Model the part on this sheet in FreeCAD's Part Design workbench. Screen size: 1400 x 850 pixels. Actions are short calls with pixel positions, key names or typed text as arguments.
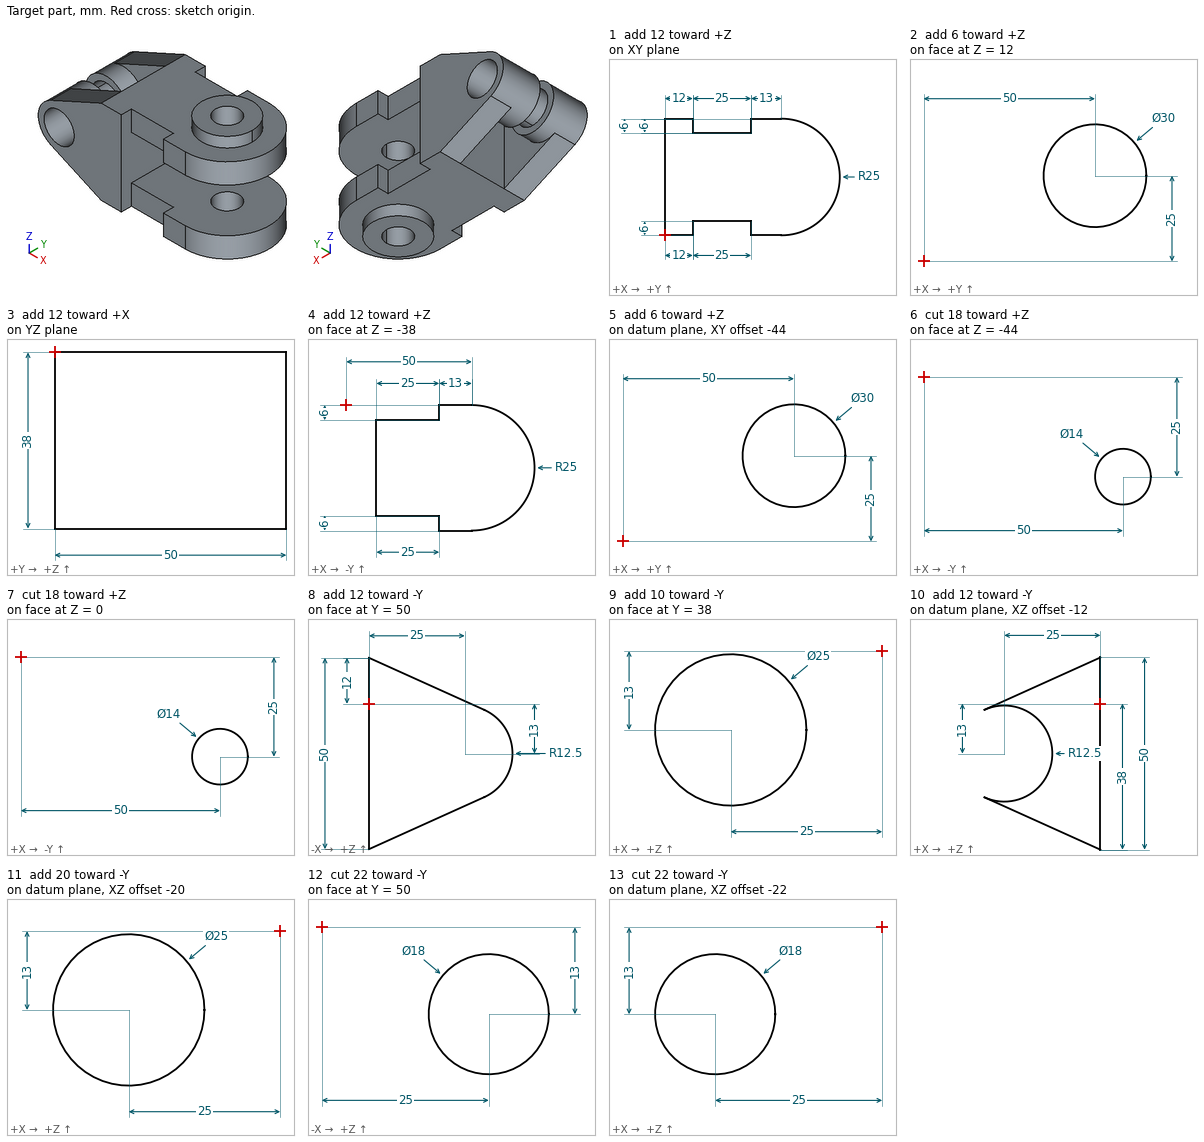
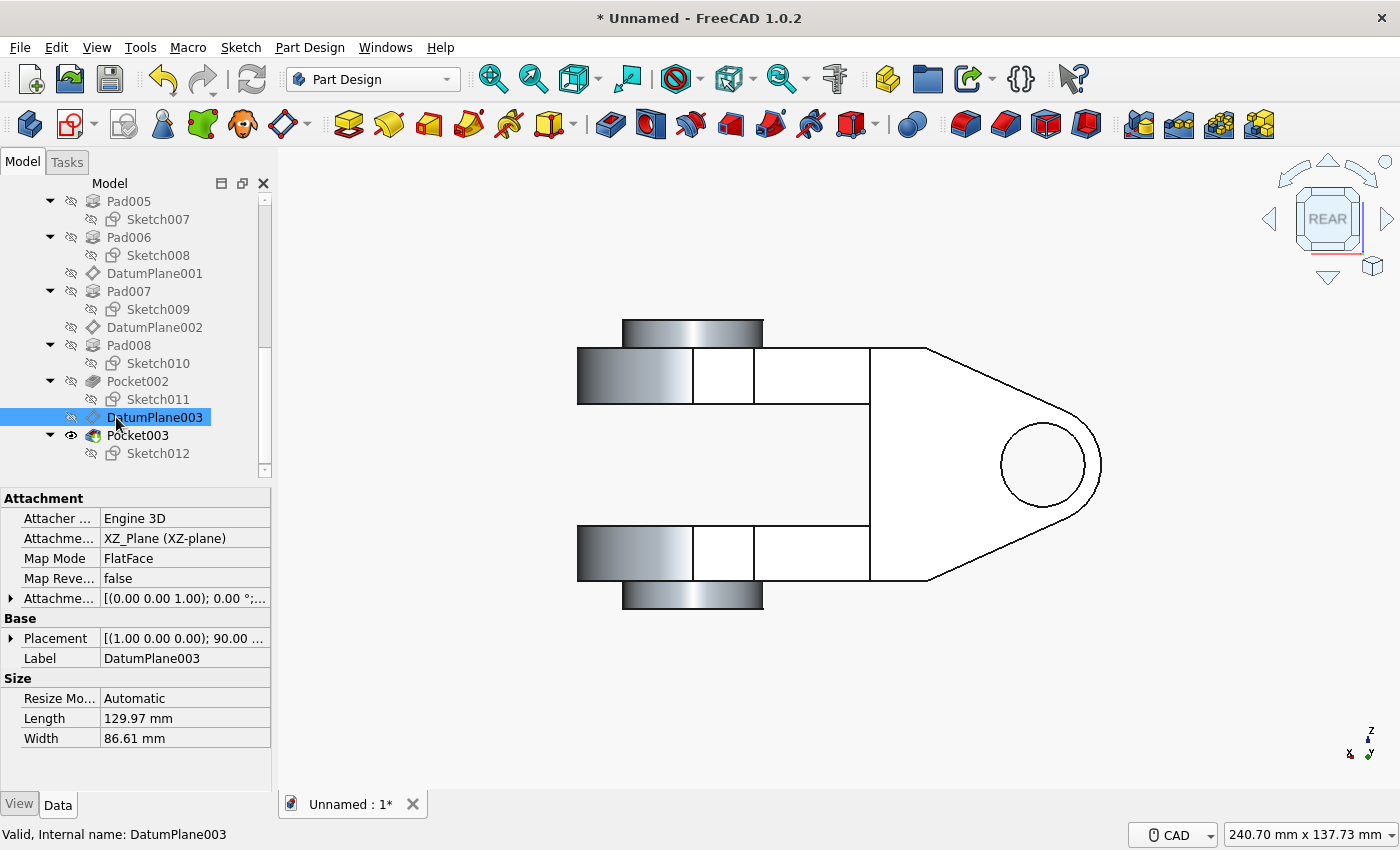
key(0)